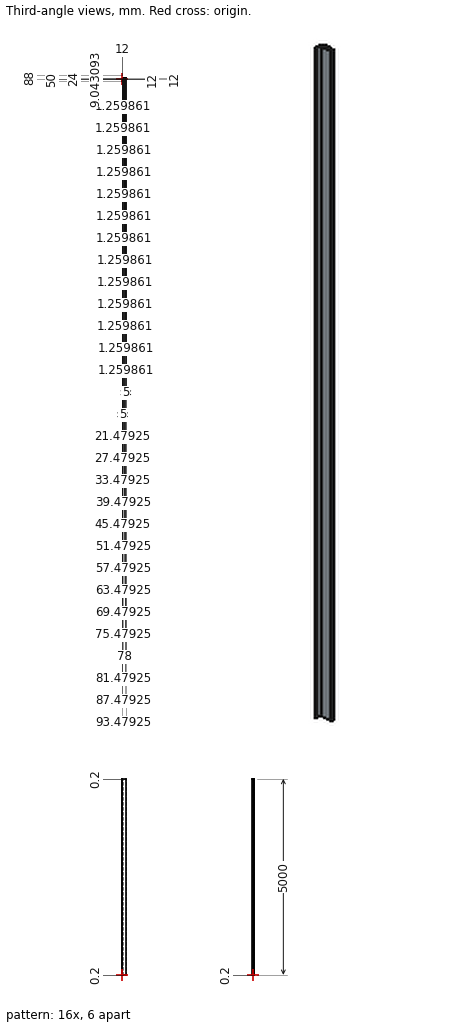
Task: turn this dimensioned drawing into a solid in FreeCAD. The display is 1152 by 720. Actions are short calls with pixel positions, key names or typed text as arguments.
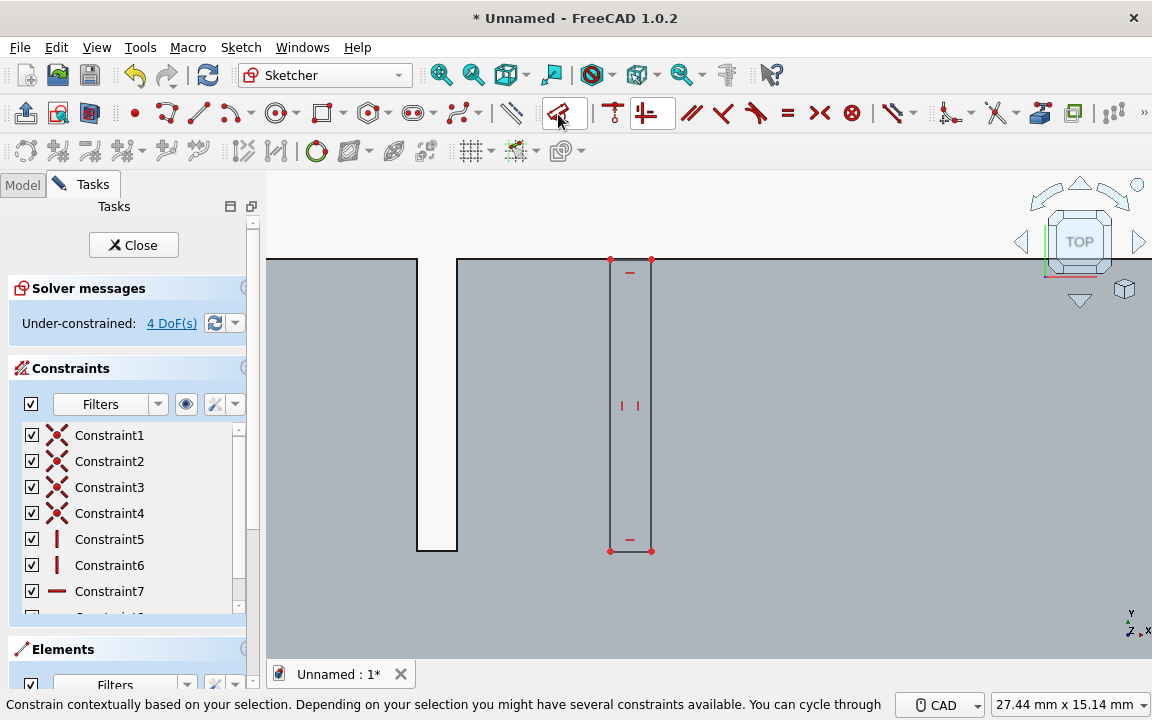
click(610, 260)
click(644, 575)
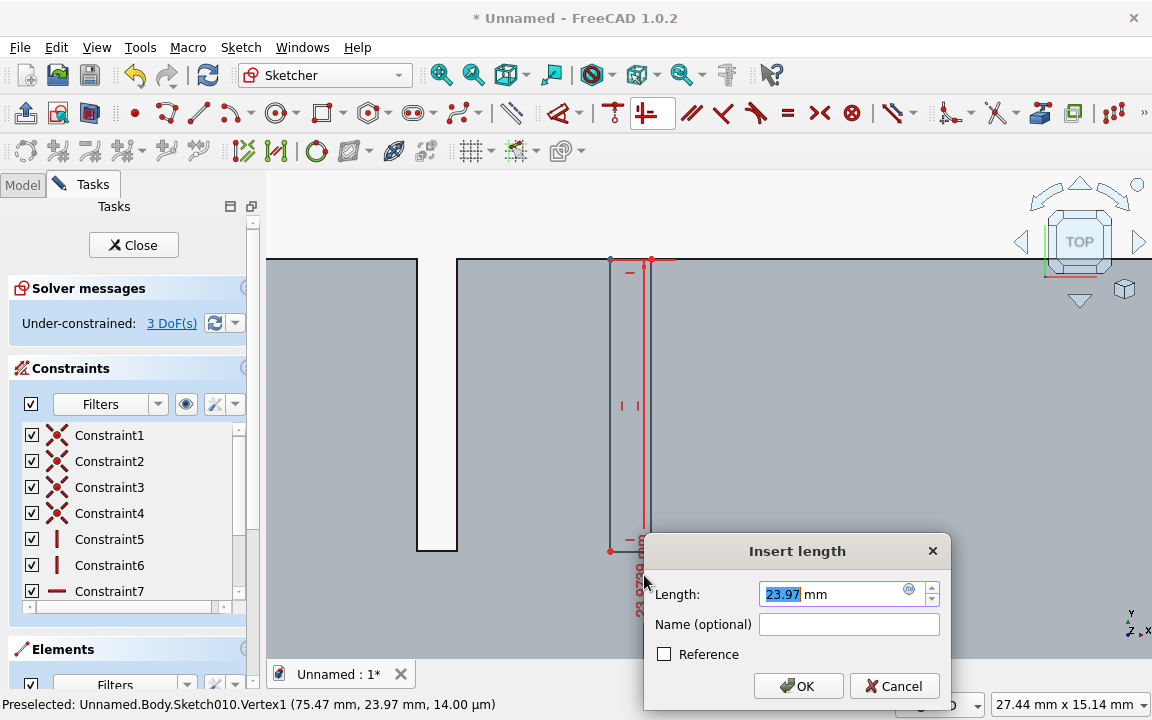
text(24)
key(Return)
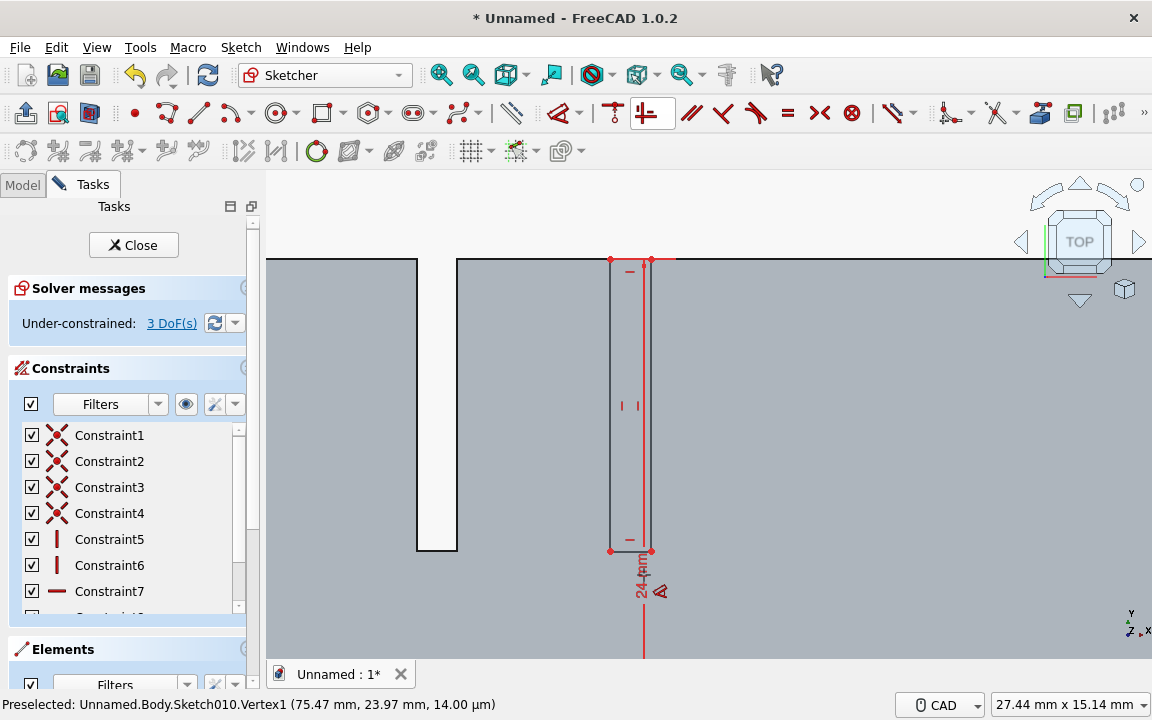
click(610, 347)
click(576, 406)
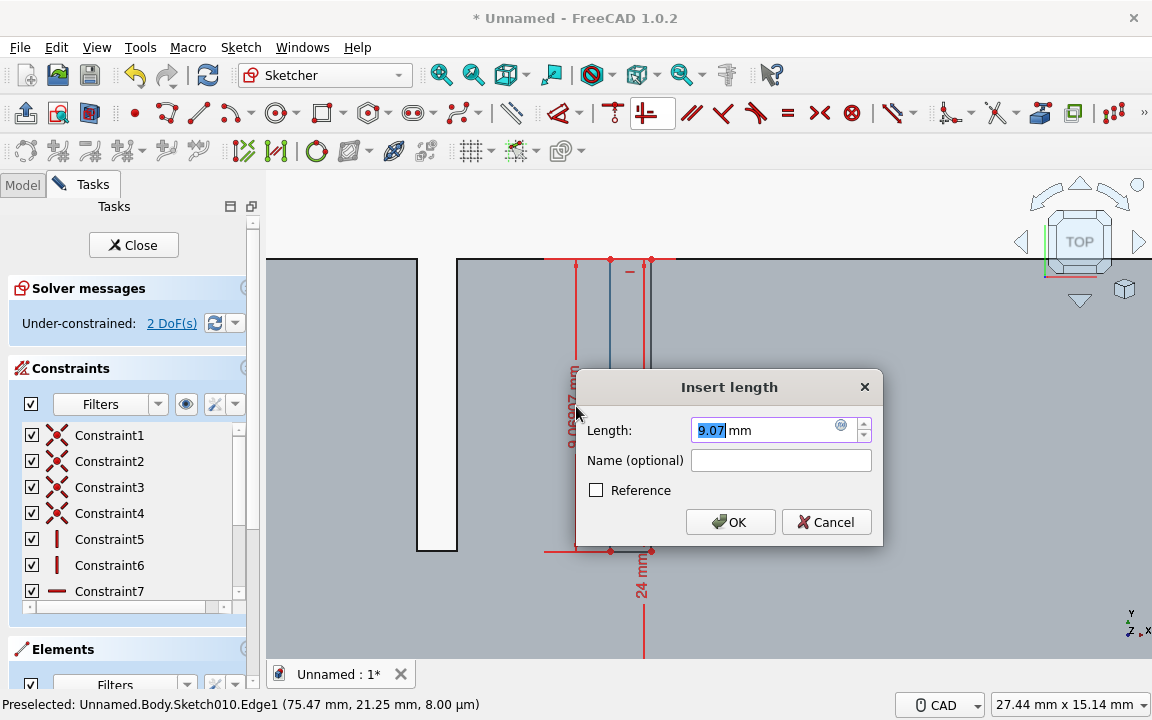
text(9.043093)
key(Return)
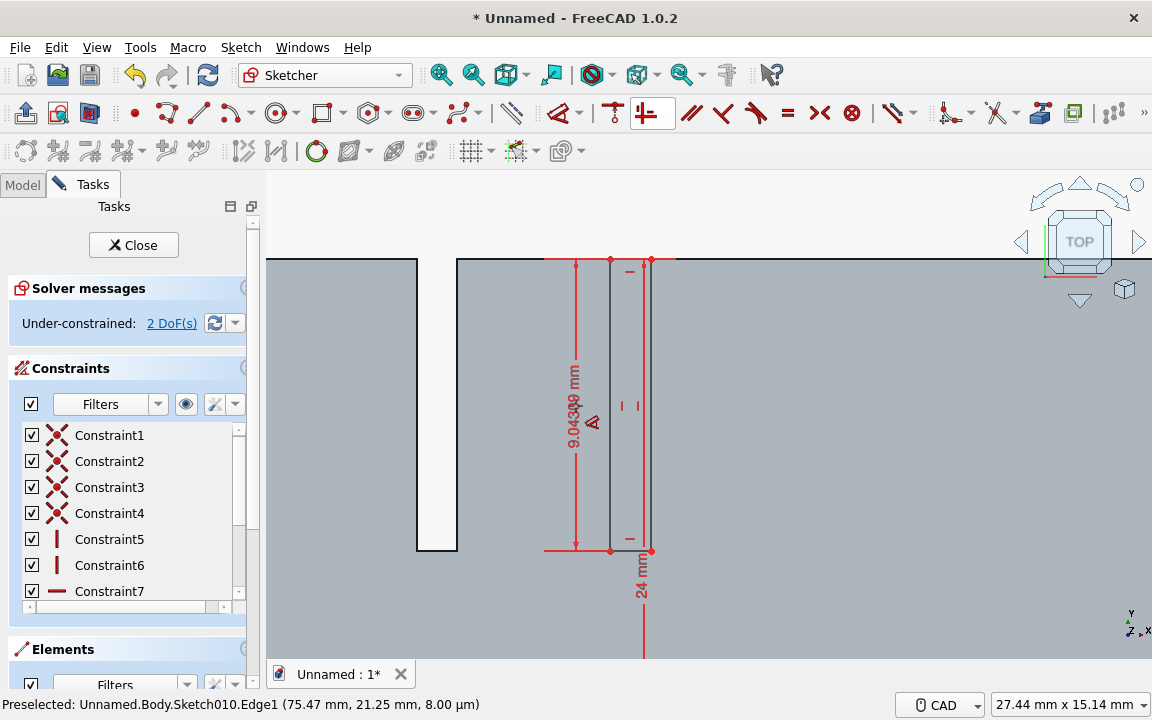
click(622, 551)
click(630, 517)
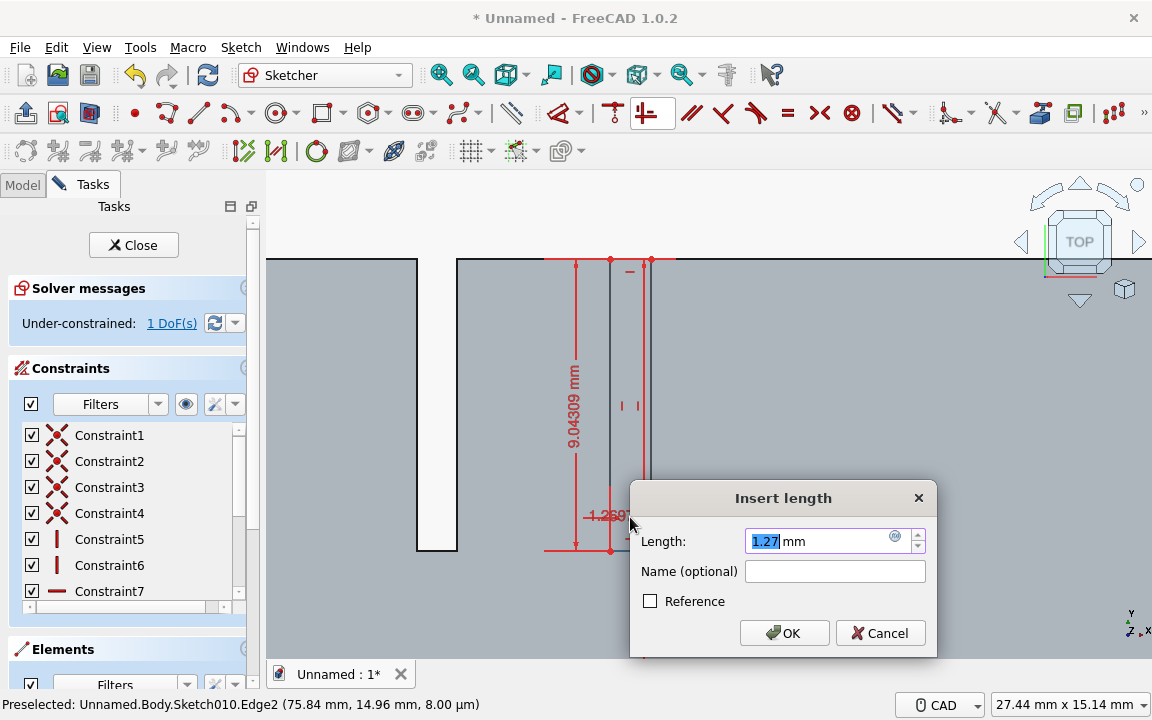
text(1.259861)
key(Return)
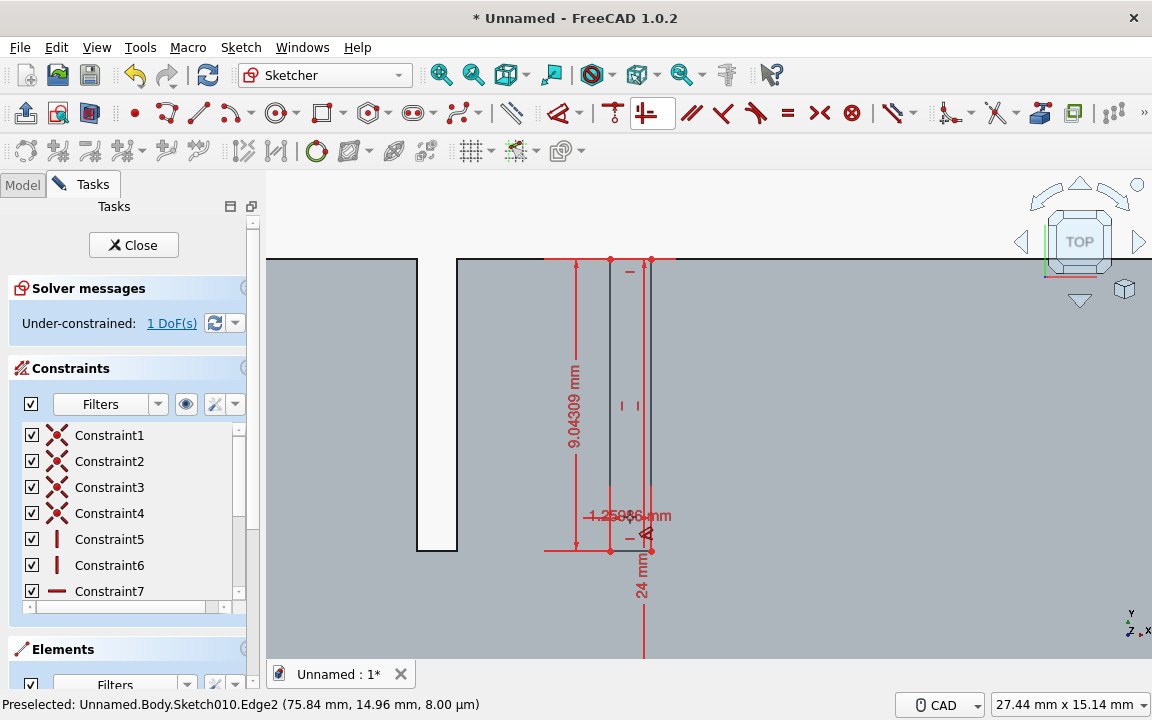
click(610, 259)
click(452, 225)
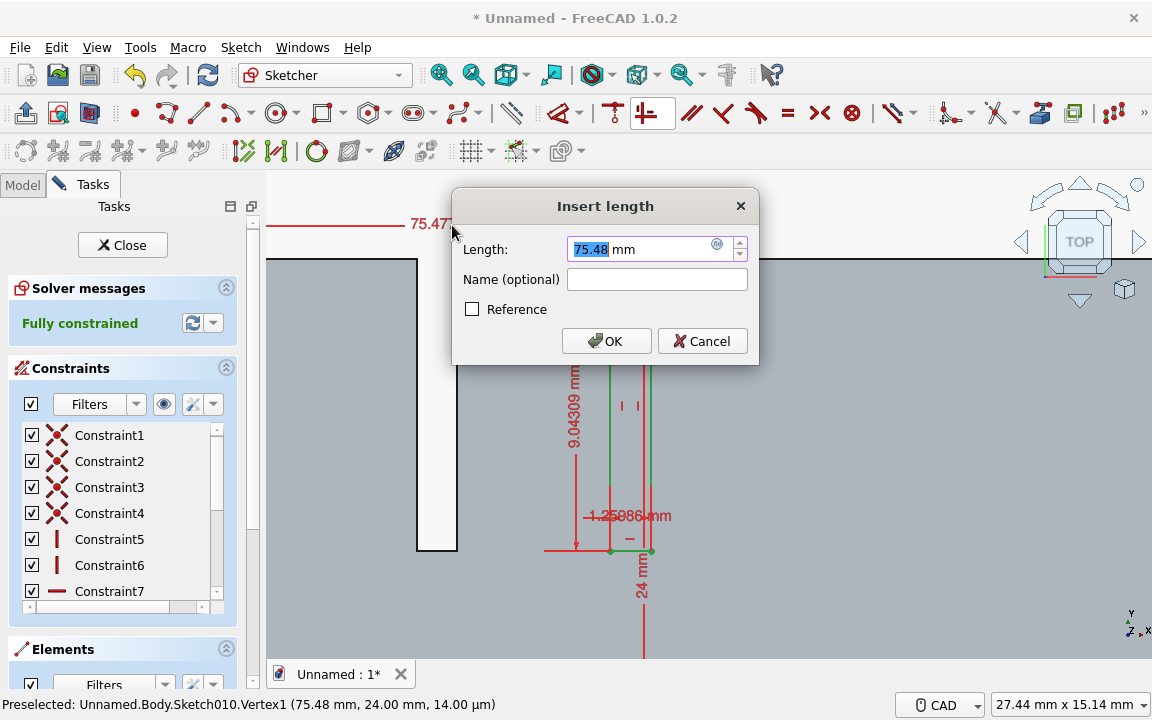
text(75.47925)
key(Return)
key(Escape)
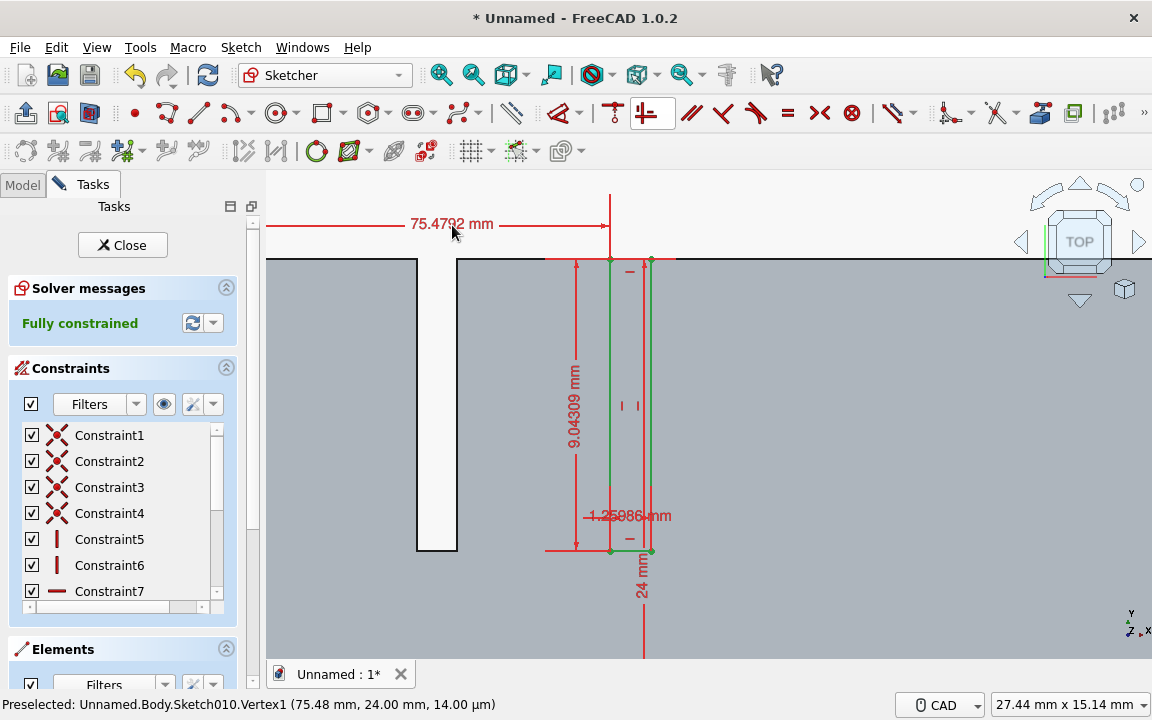
click(123, 245)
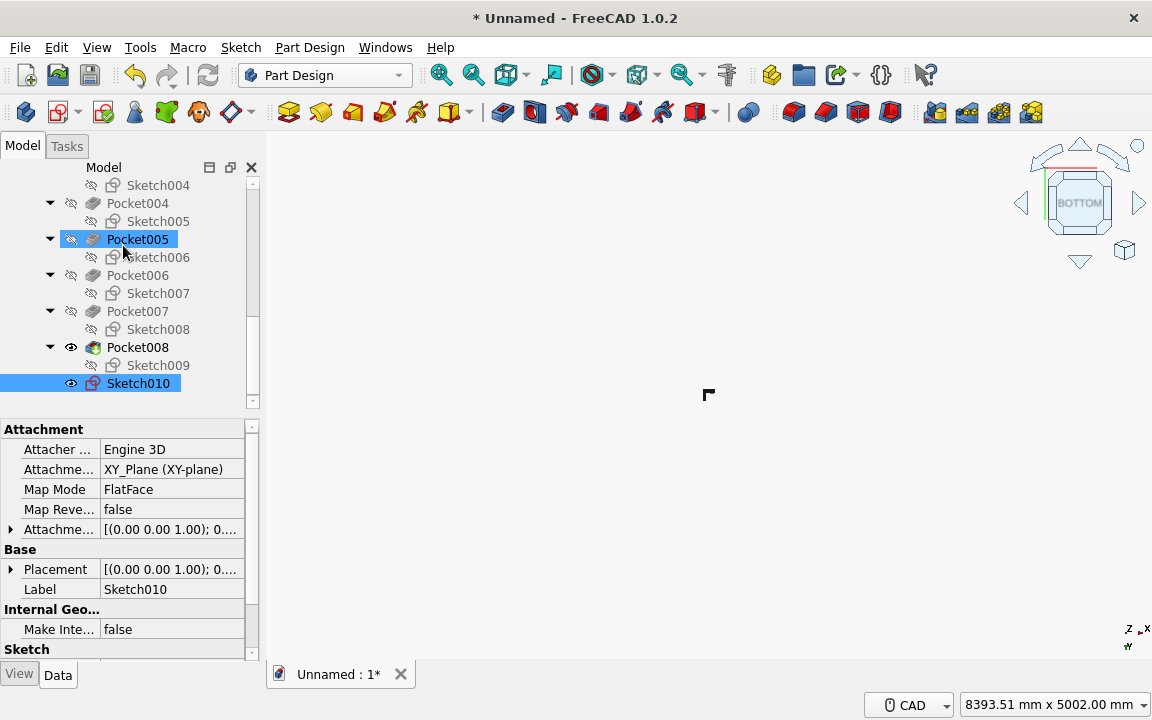
click(504, 112)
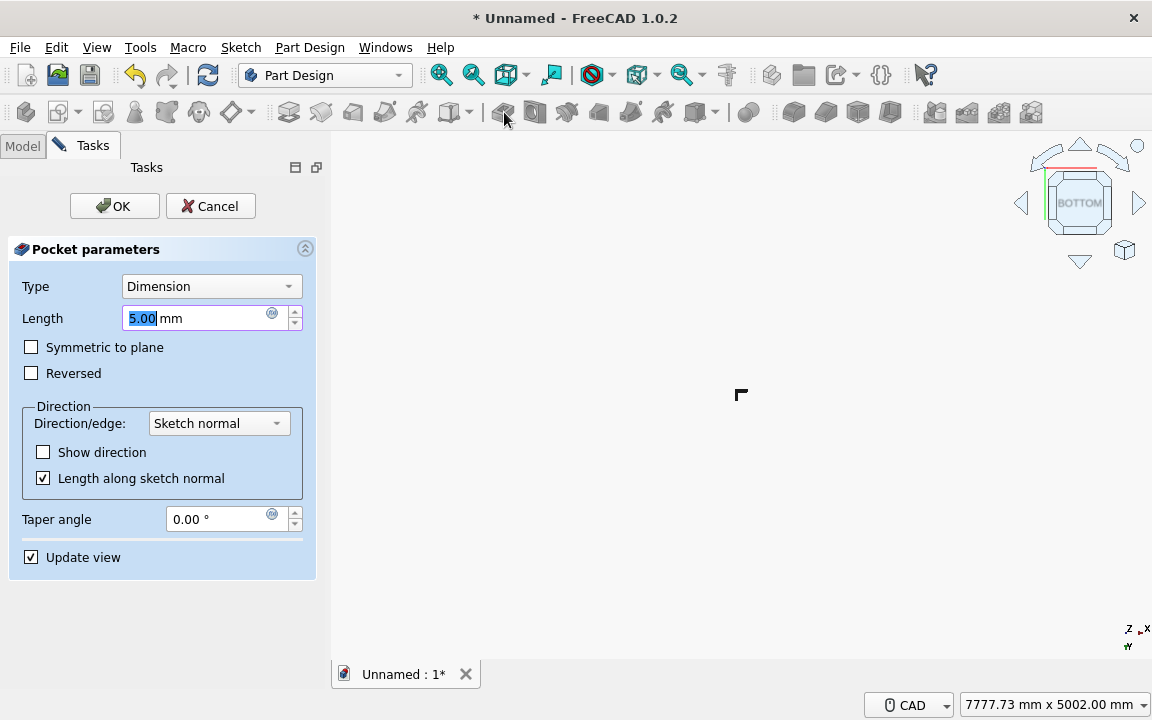
text(0.2)
key(Tab)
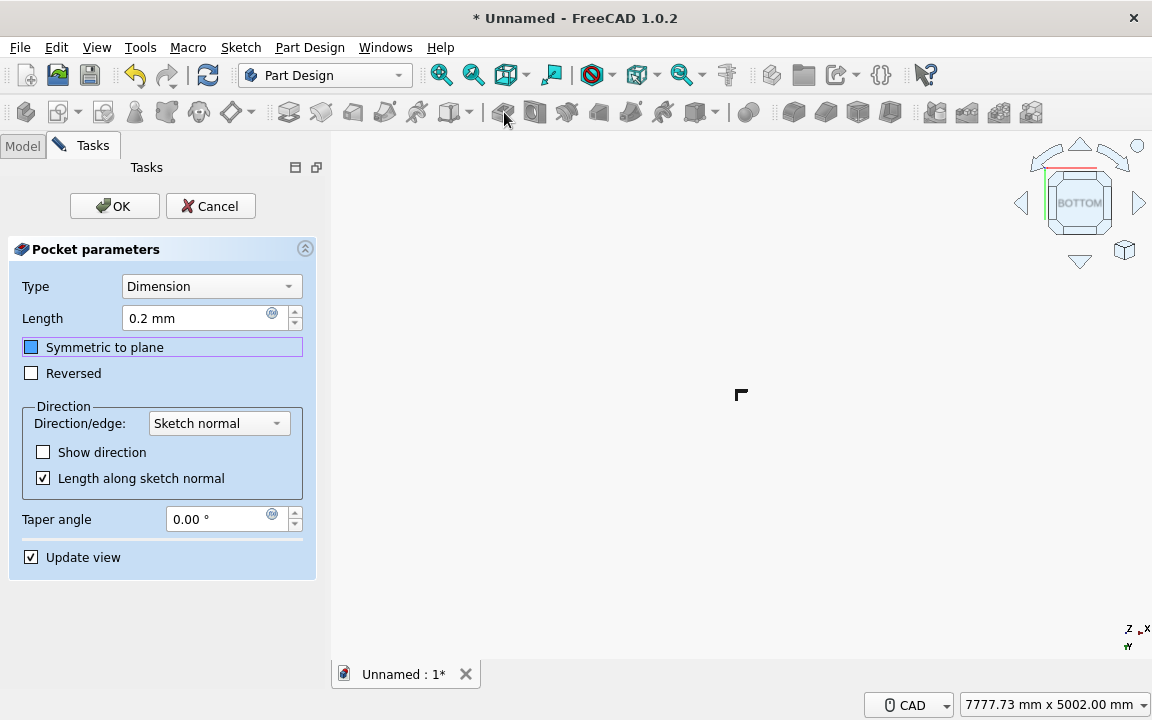
click(30, 373)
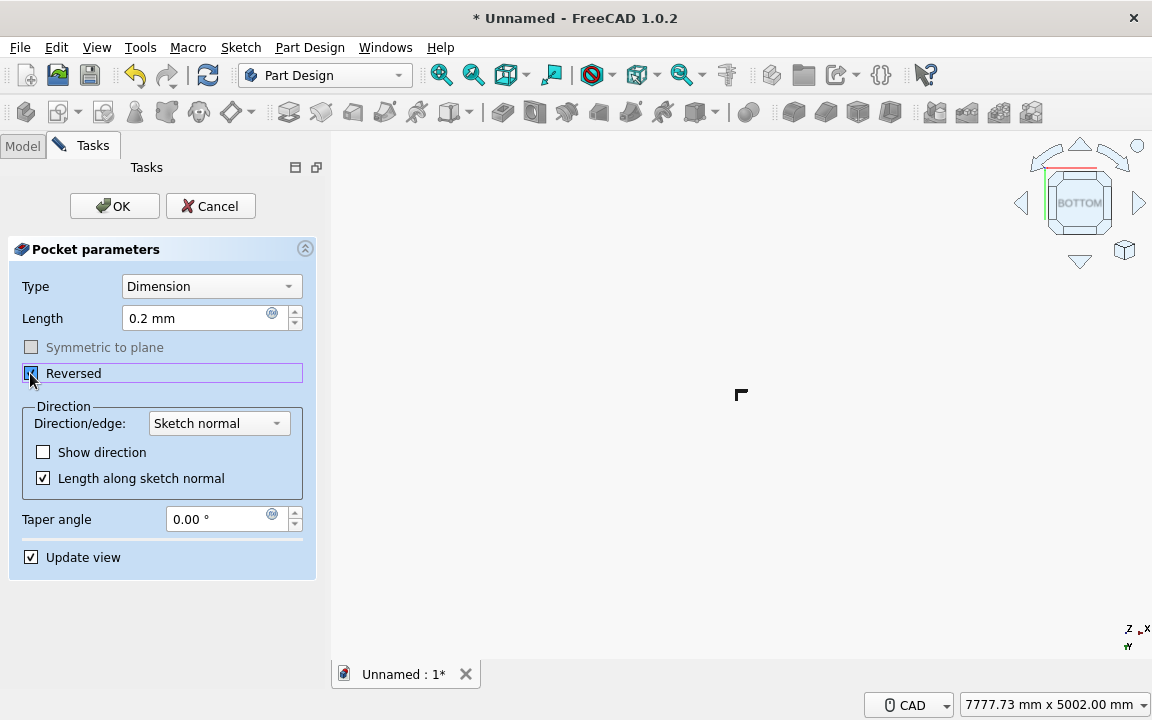
click(115, 206)